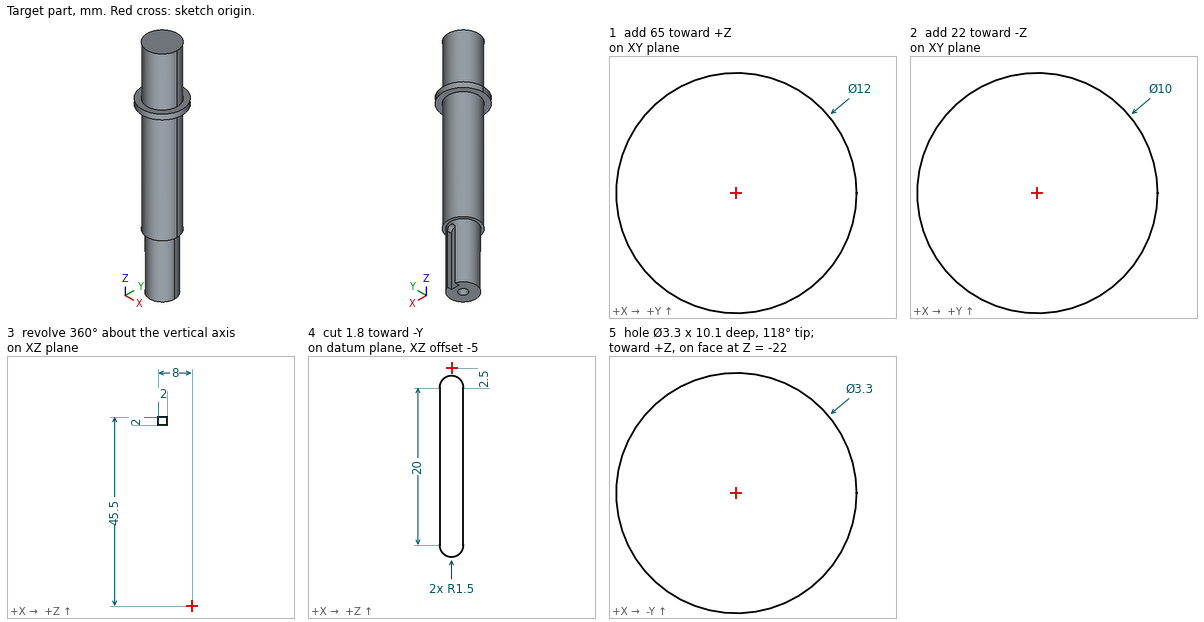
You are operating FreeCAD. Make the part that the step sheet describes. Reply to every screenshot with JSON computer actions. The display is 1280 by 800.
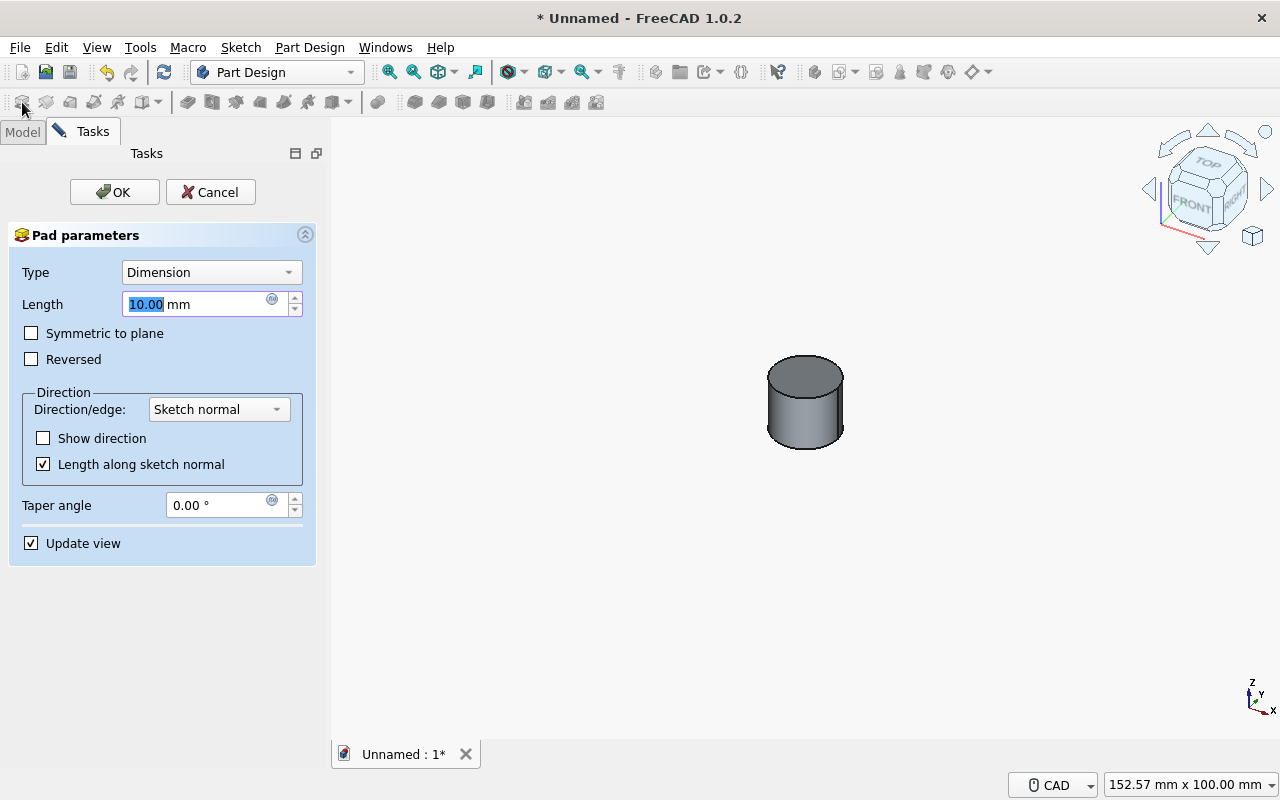
{"action": "type", "text": "65"}
{"action": "key", "text": "Tab"}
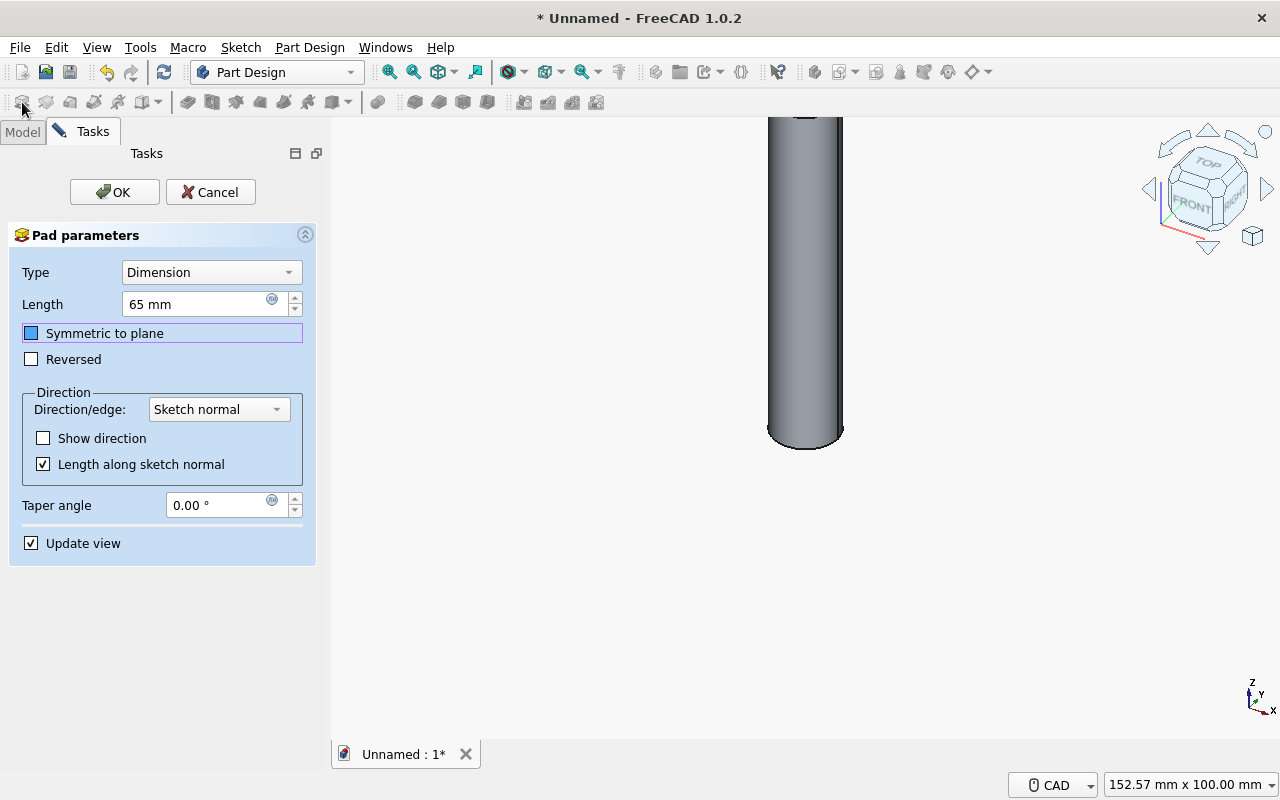
{"action": "left_click", "coordinate": [115, 192]}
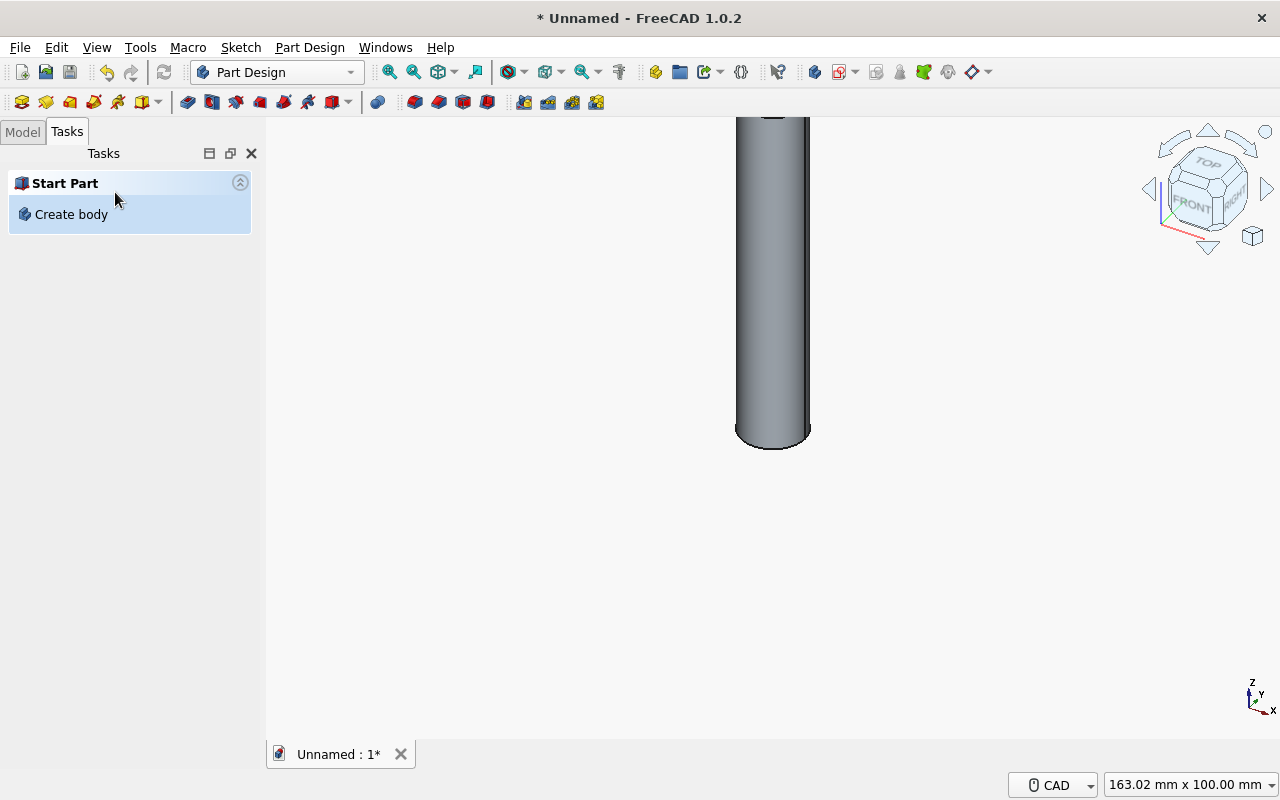
{"action": "left_click", "coordinate": [390, 72]}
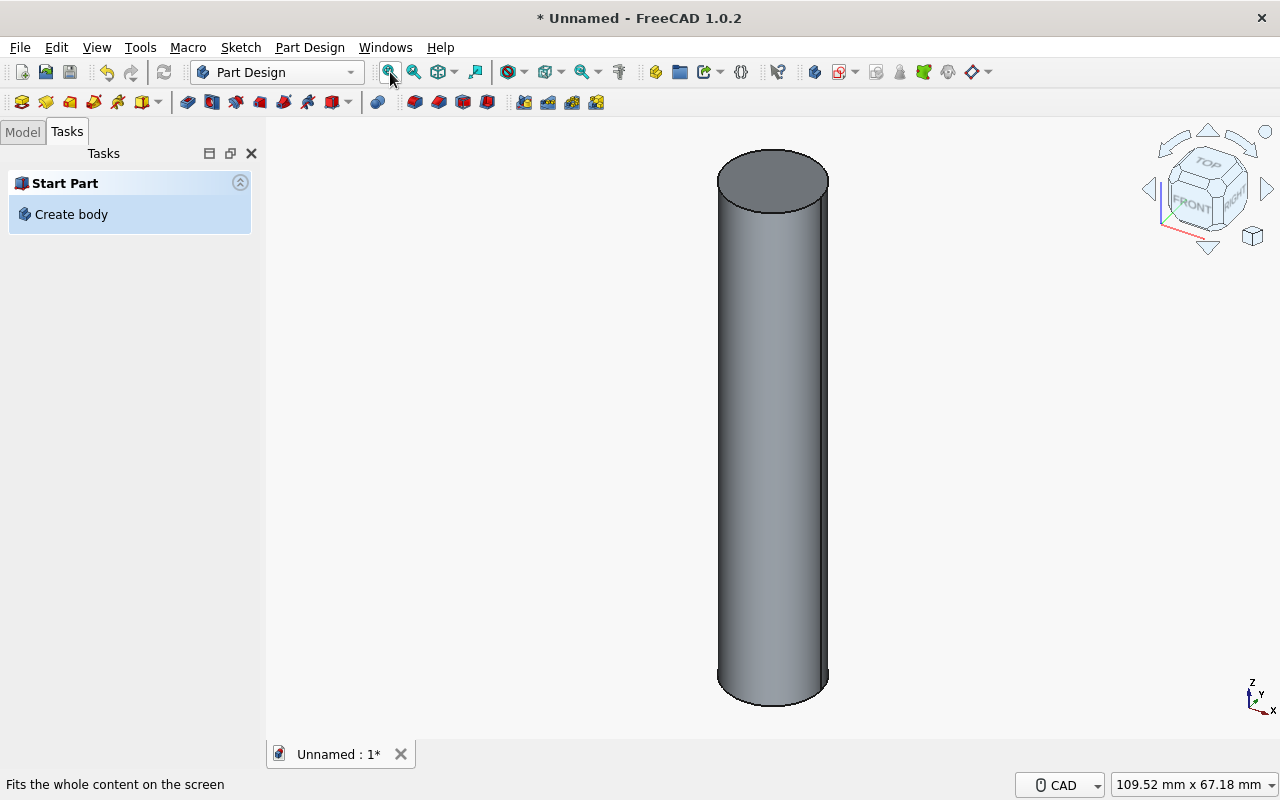
{"action": "left_click", "coordinate": [840, 72]}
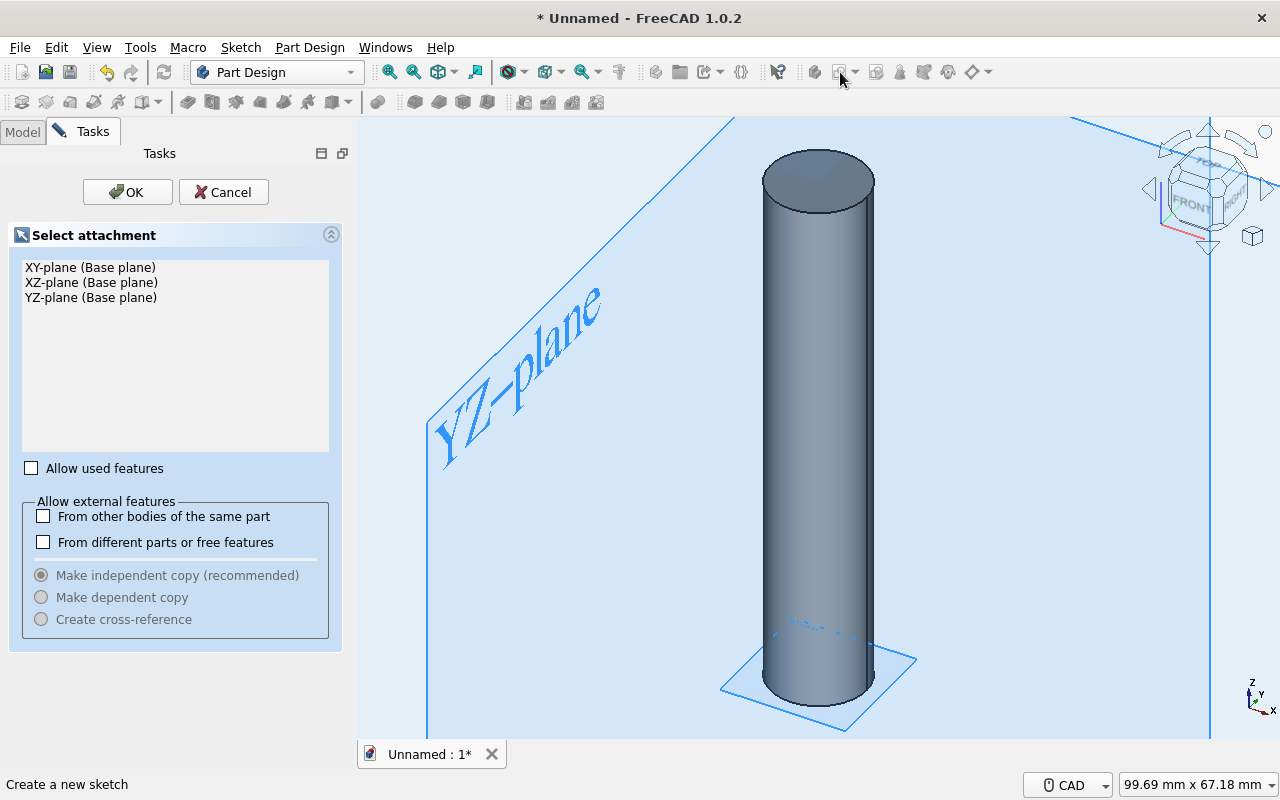
{"action": "left_click", "coordinate": [82, 268]}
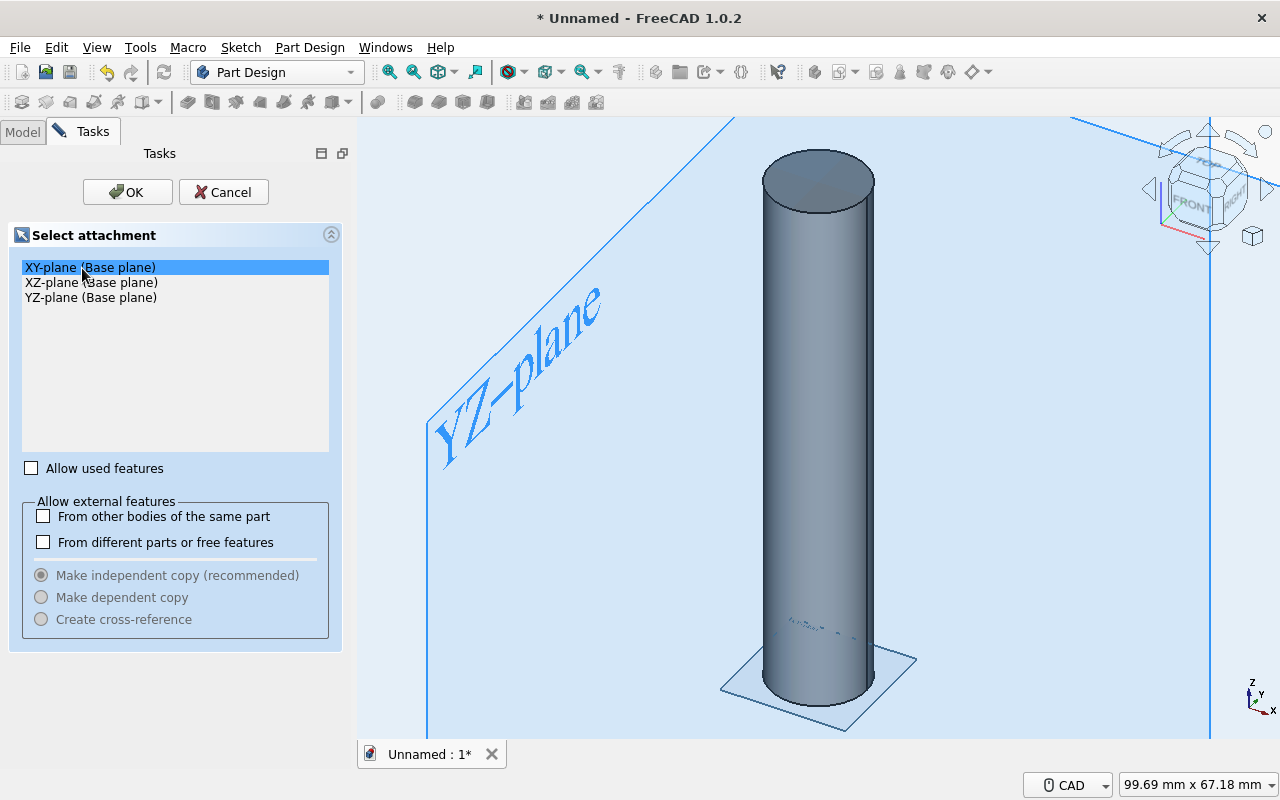
{"action": "left_click", "coordinate": [128, 192]}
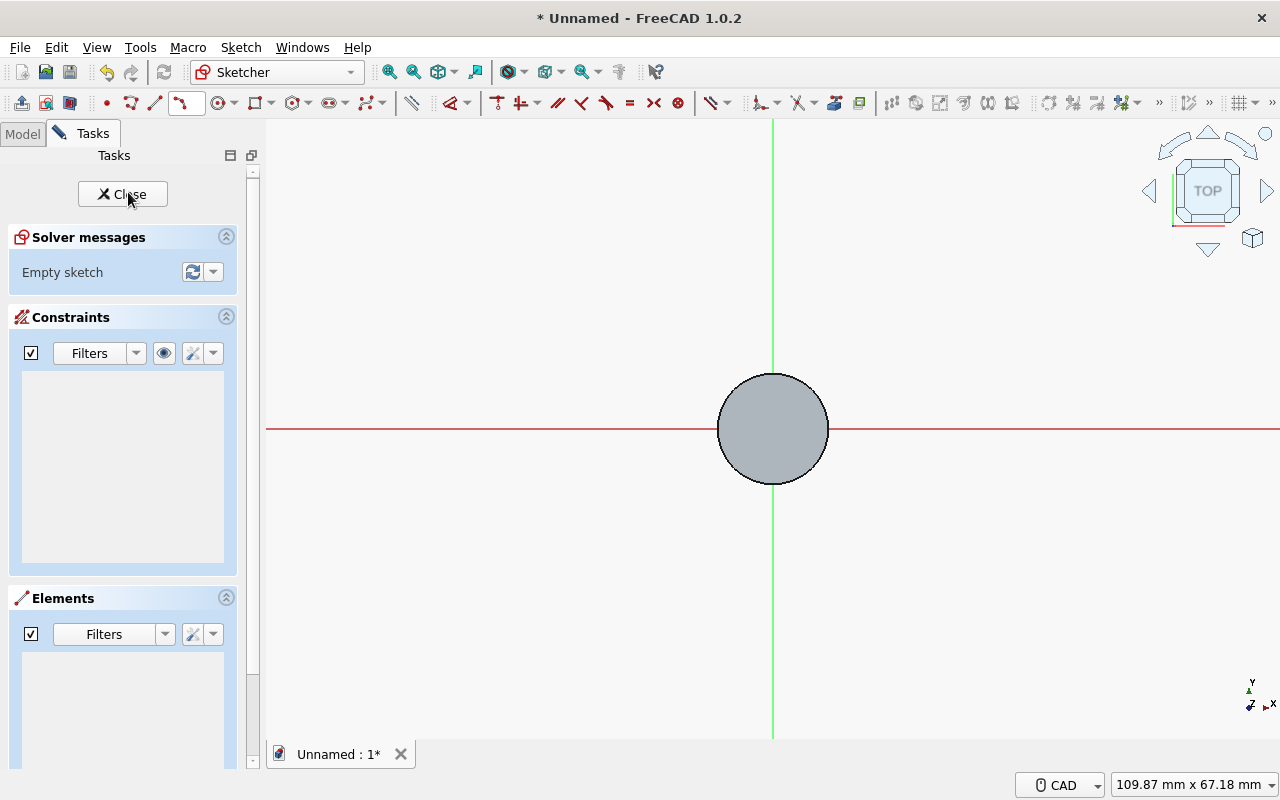
{"action": "left_click", "coordinate": [70, 104]}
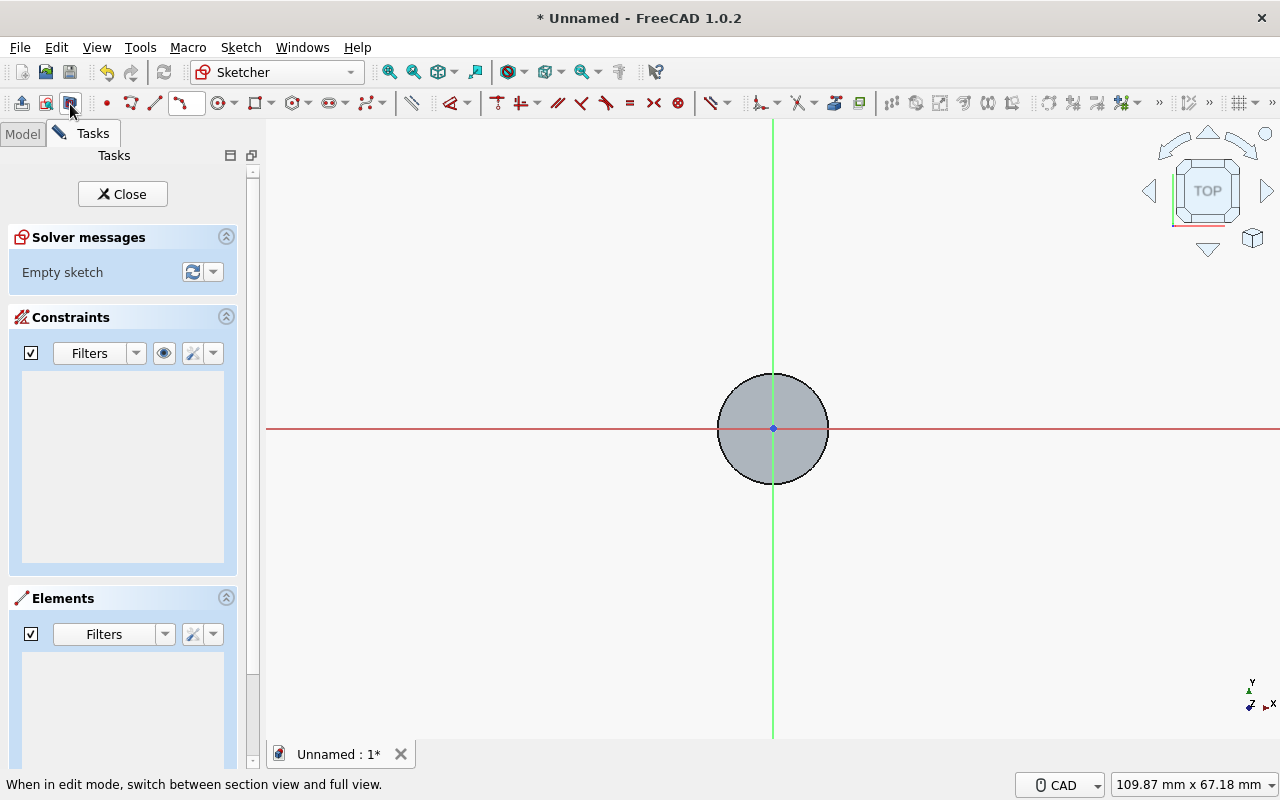
{"action": "scroll", "coordinate": [795, 429], "scroll_direction": "up", "scroll_amount": 7}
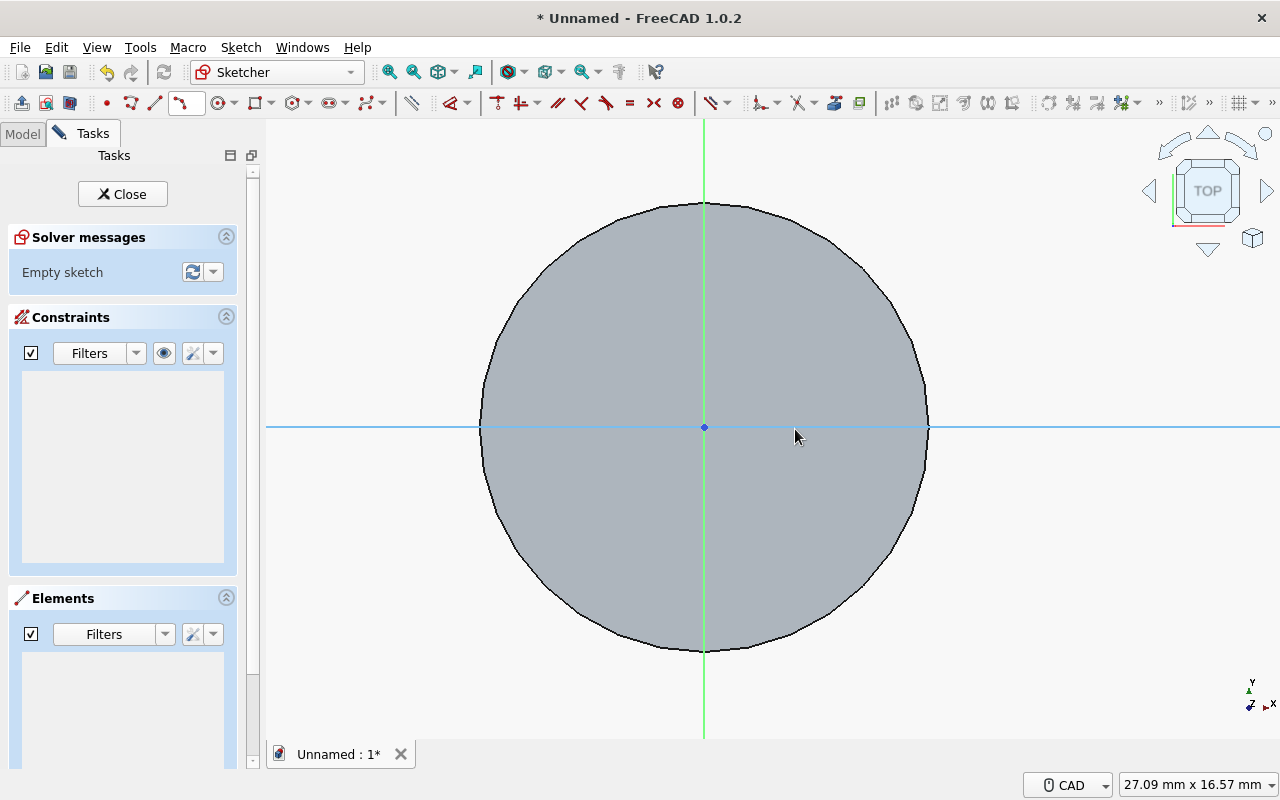
{"action": "left_click", "coordinate": [218, 104]}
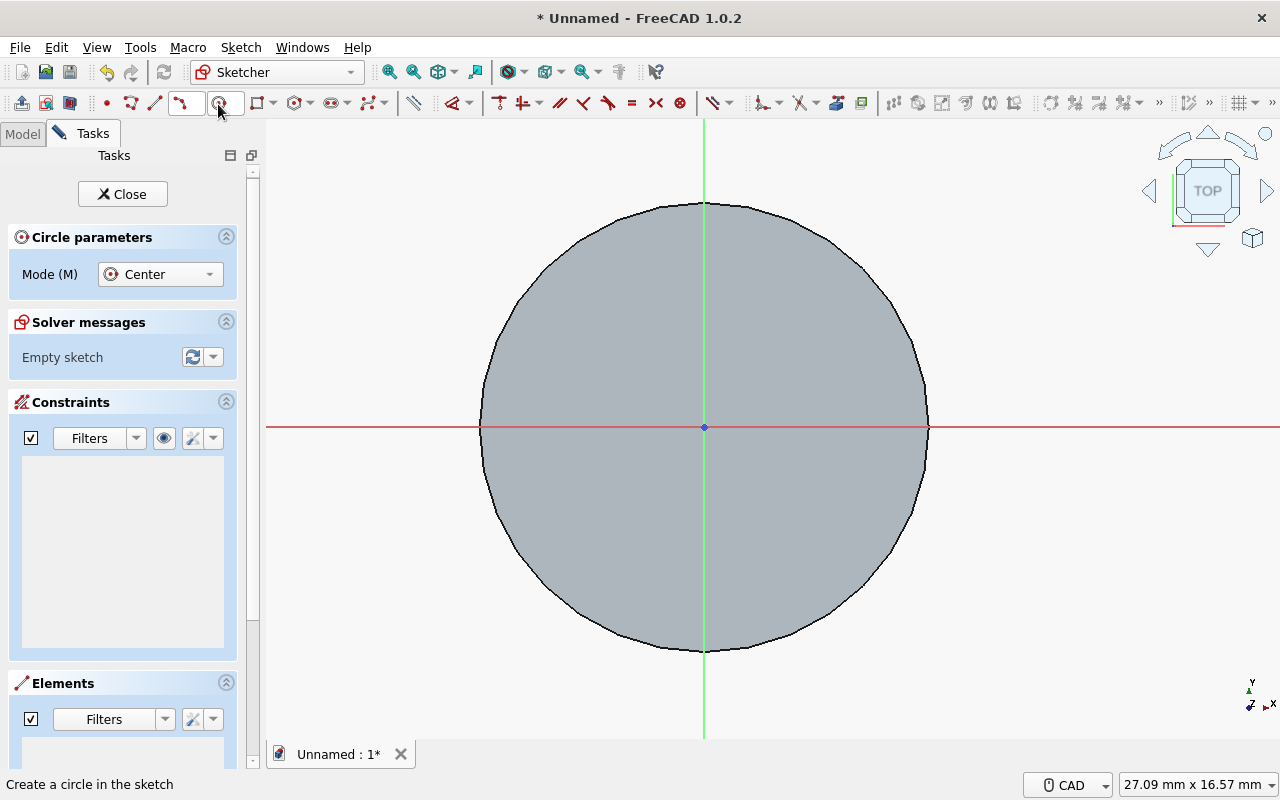
{"action": "left_click", "coordinate": [704, 427]}
{"action": "mouse_move", "coordinate": [837, 295]}